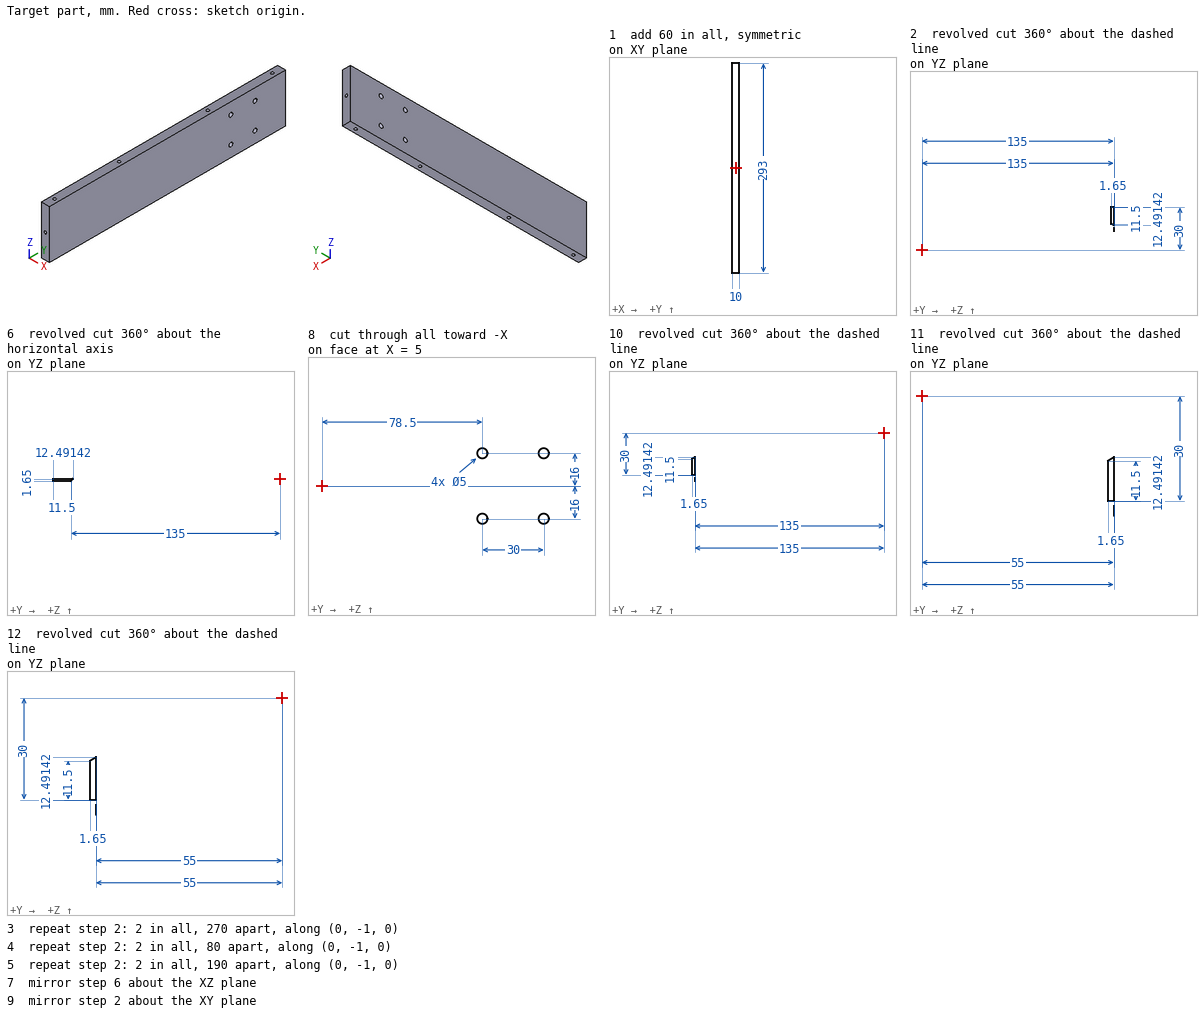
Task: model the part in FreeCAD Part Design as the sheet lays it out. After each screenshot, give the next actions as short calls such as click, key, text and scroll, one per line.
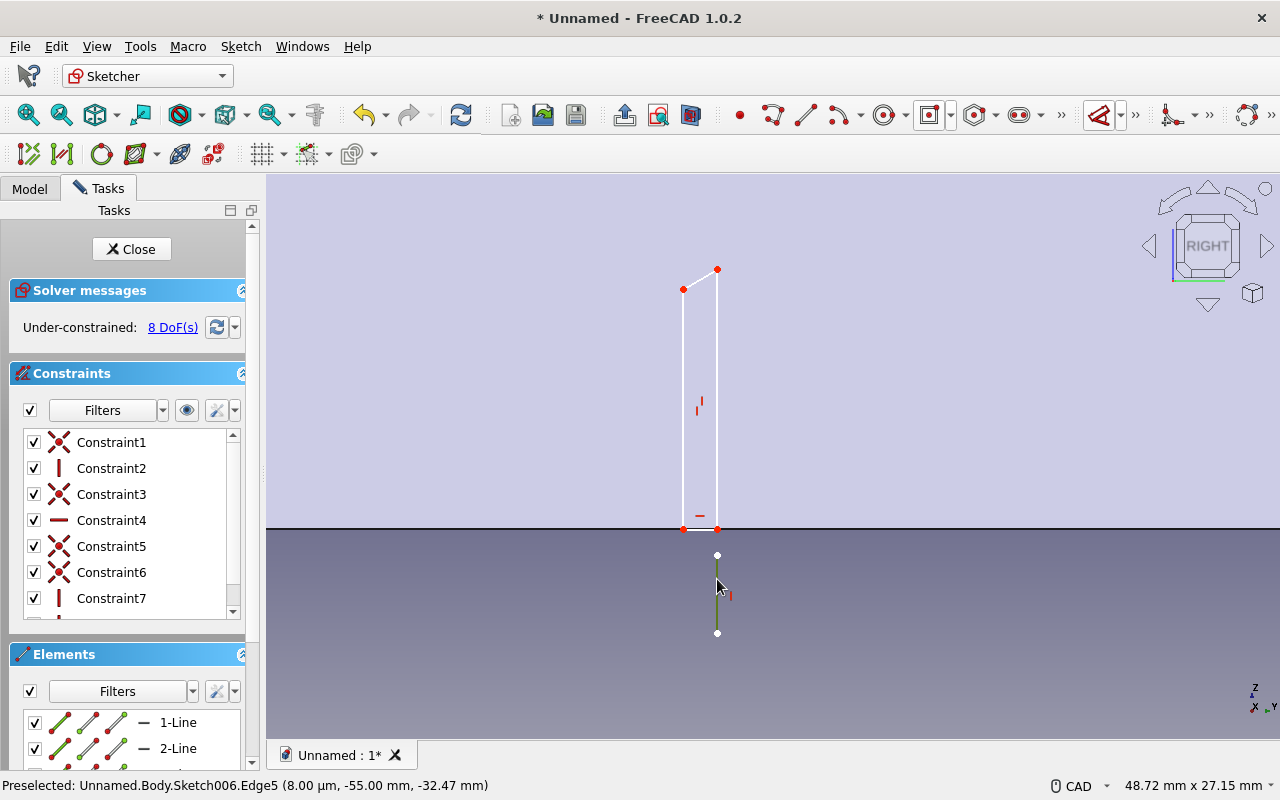
key(g)
key(n)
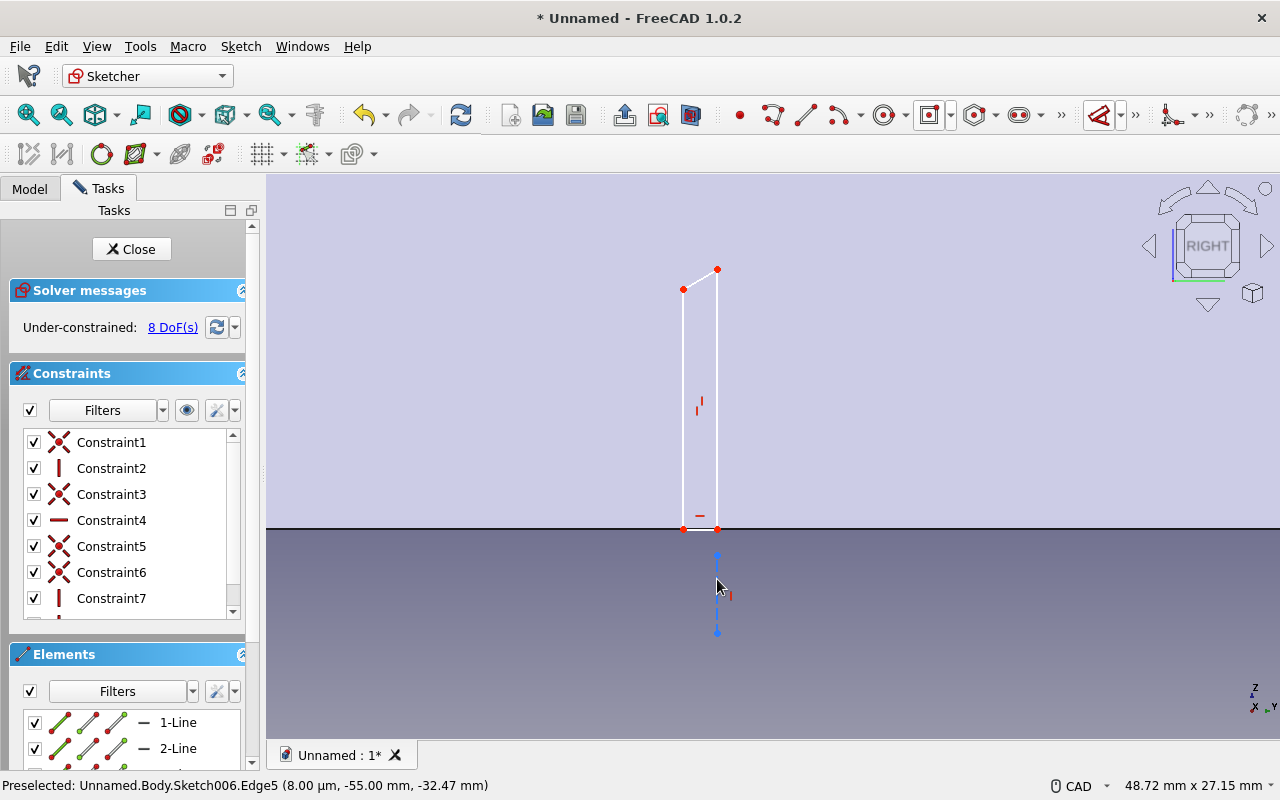
click(717, 270)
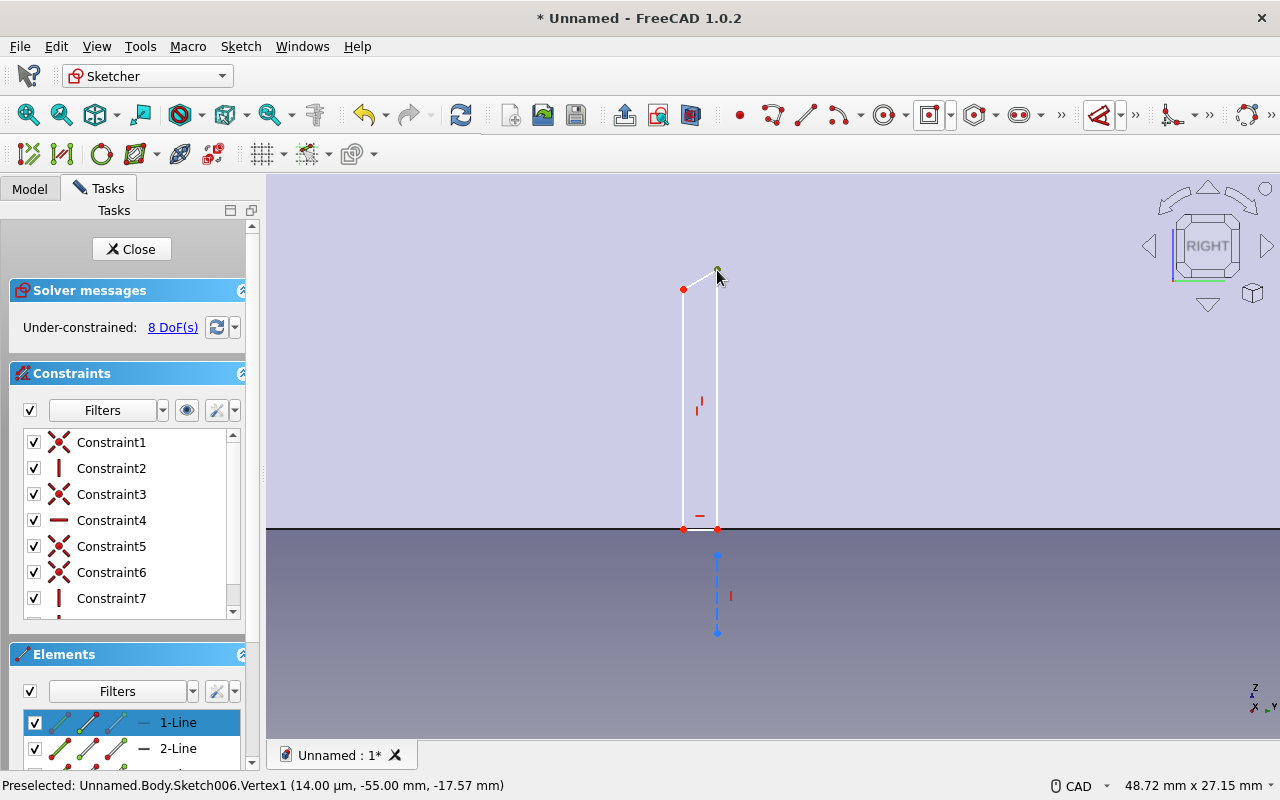
click(1120, 116)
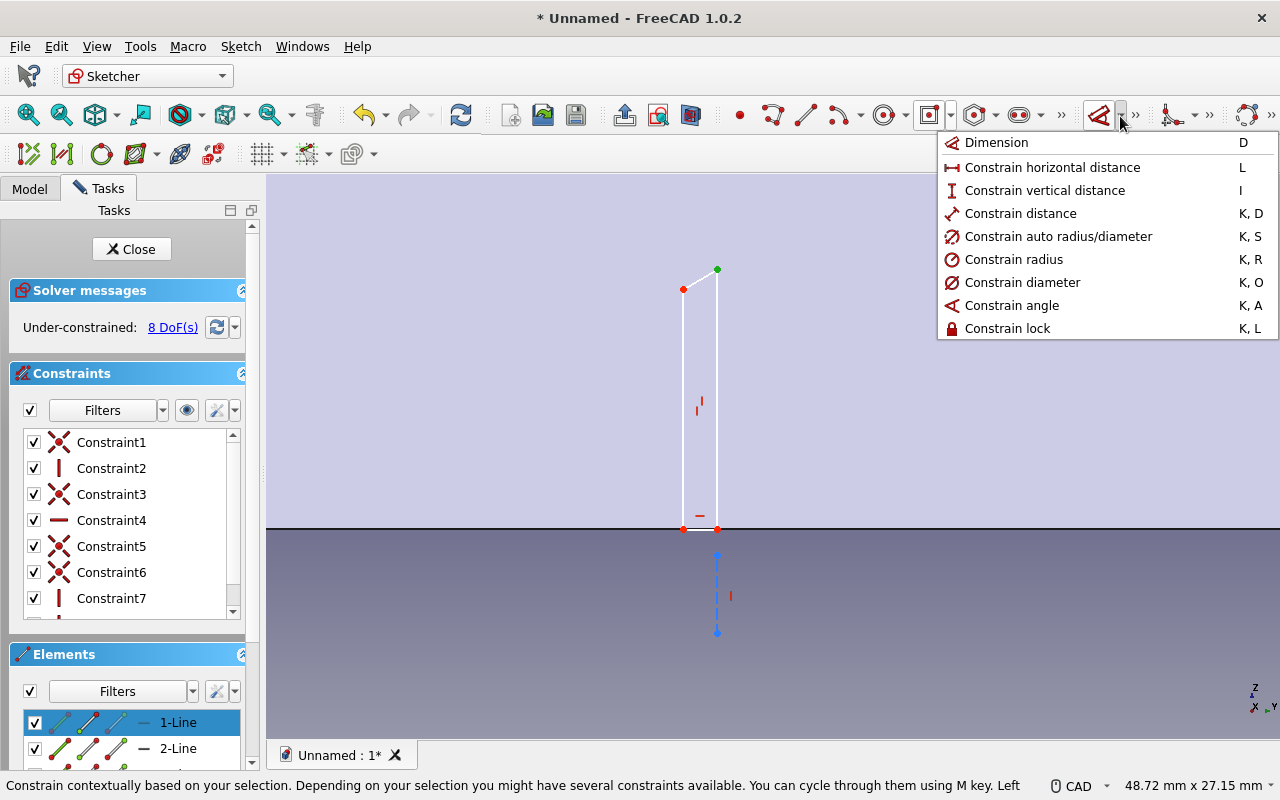
click(1108, 168)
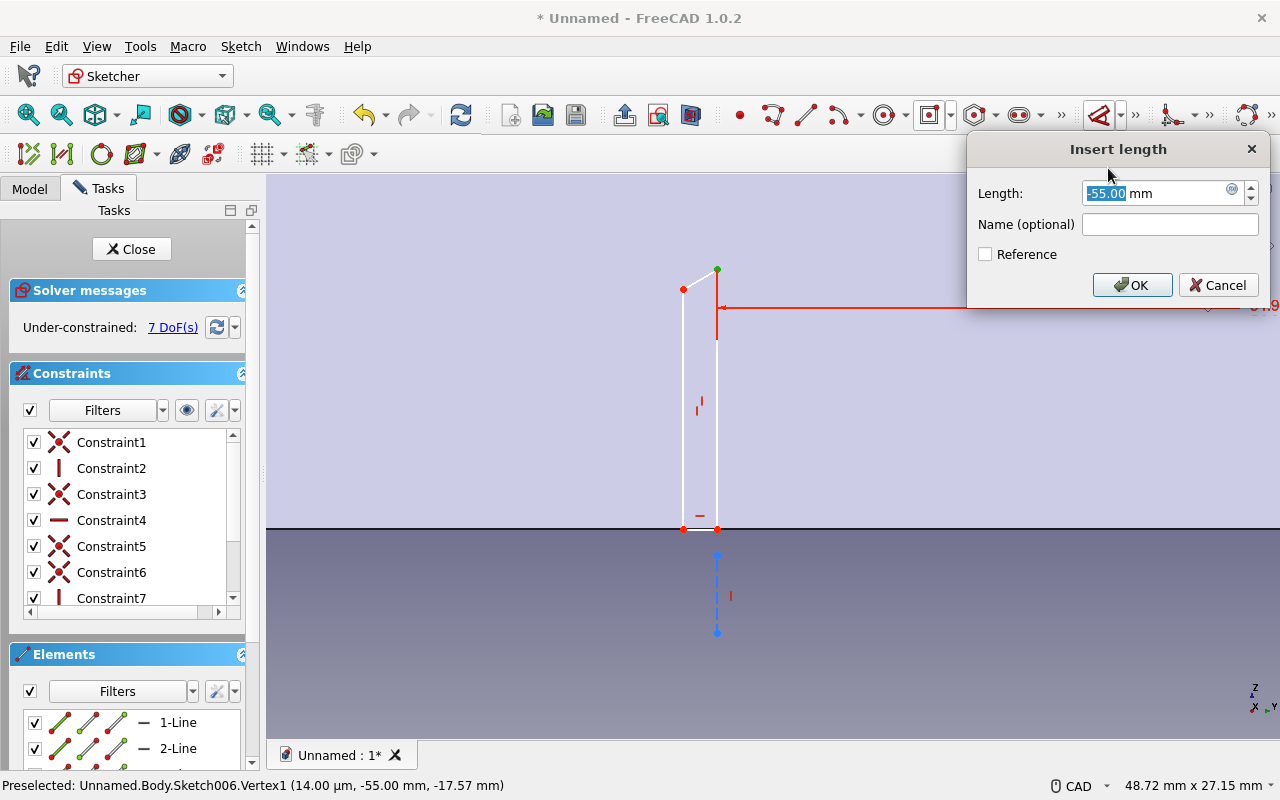
text(-55)
key(Return)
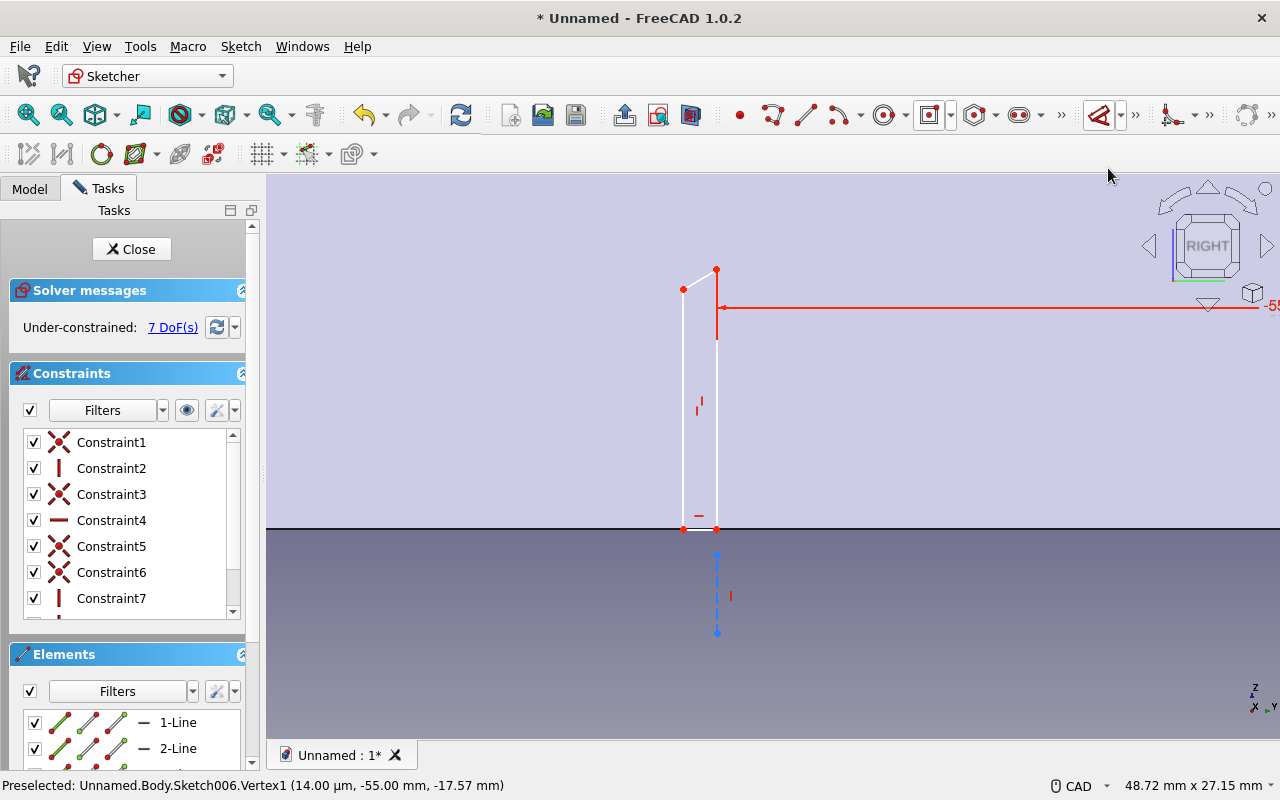
click(683, 530)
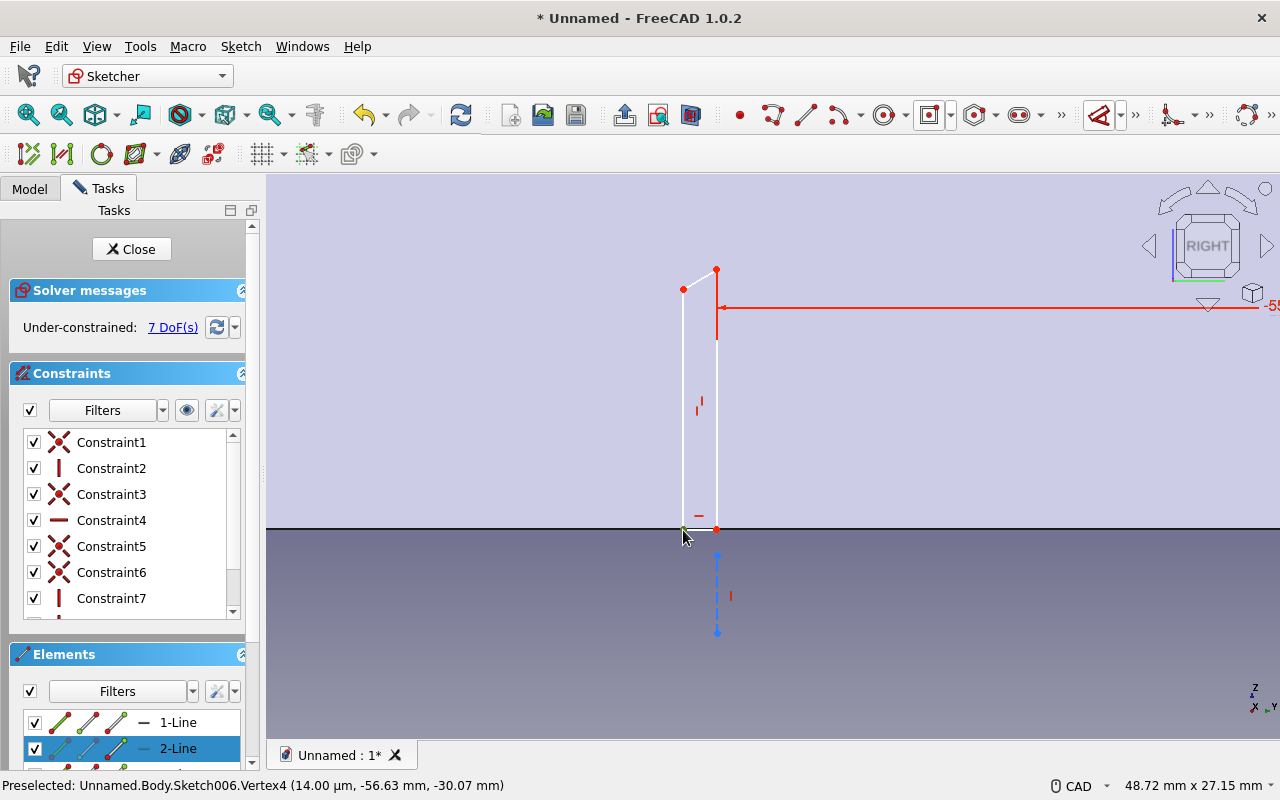
click(1120, 116)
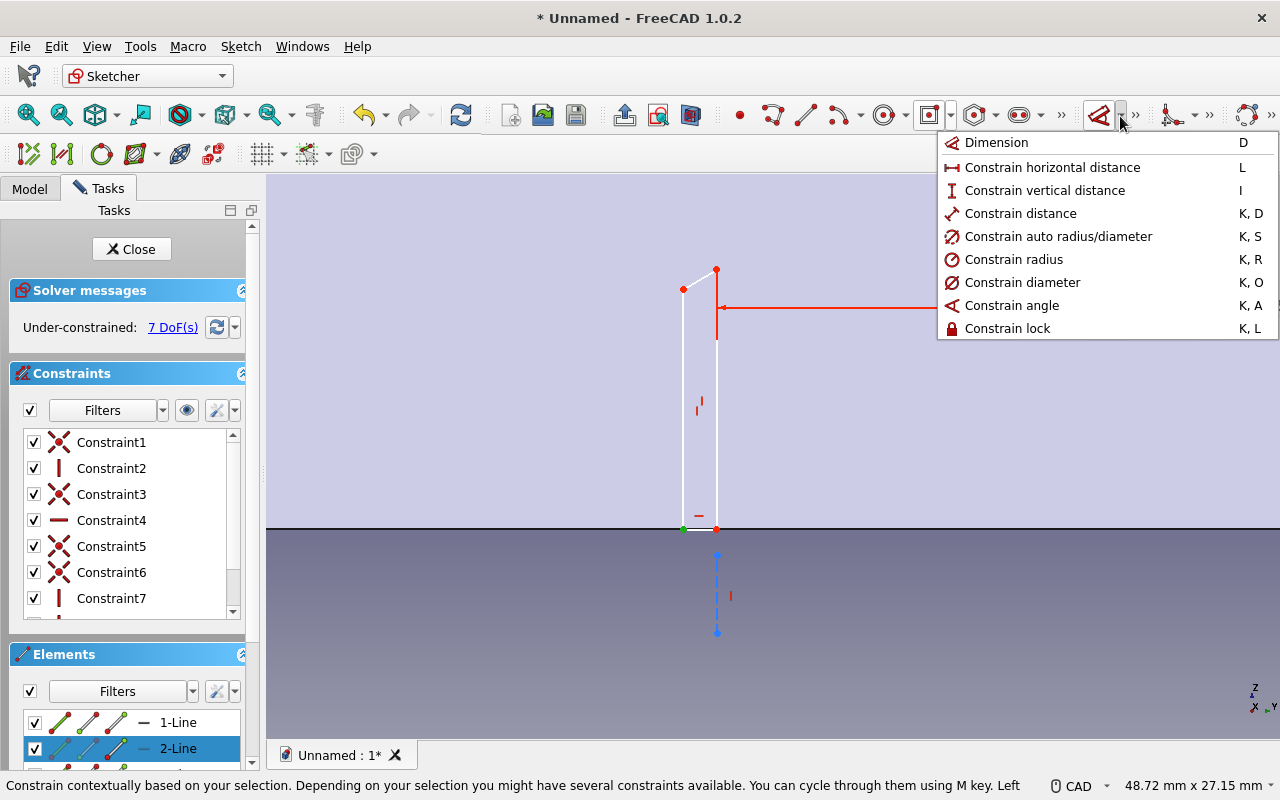
click(1108, 190)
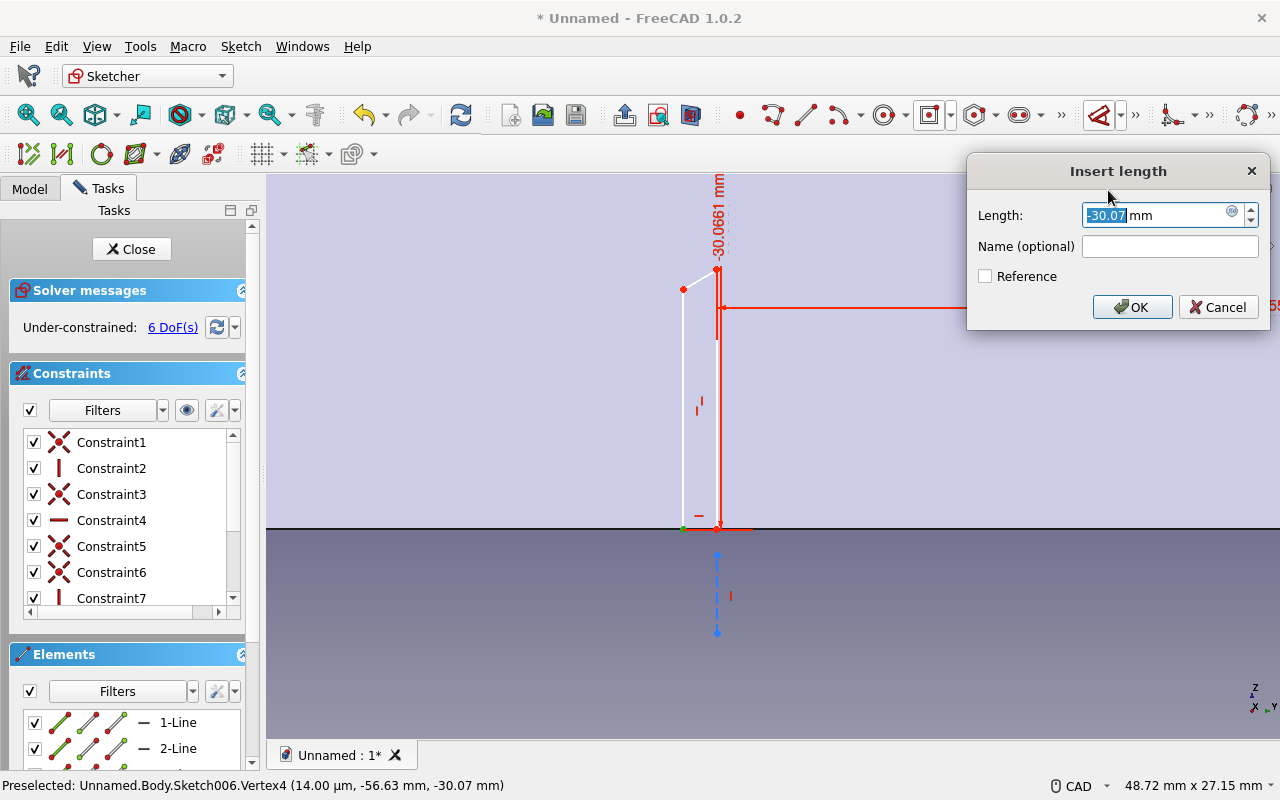
text(-30)
key(Return)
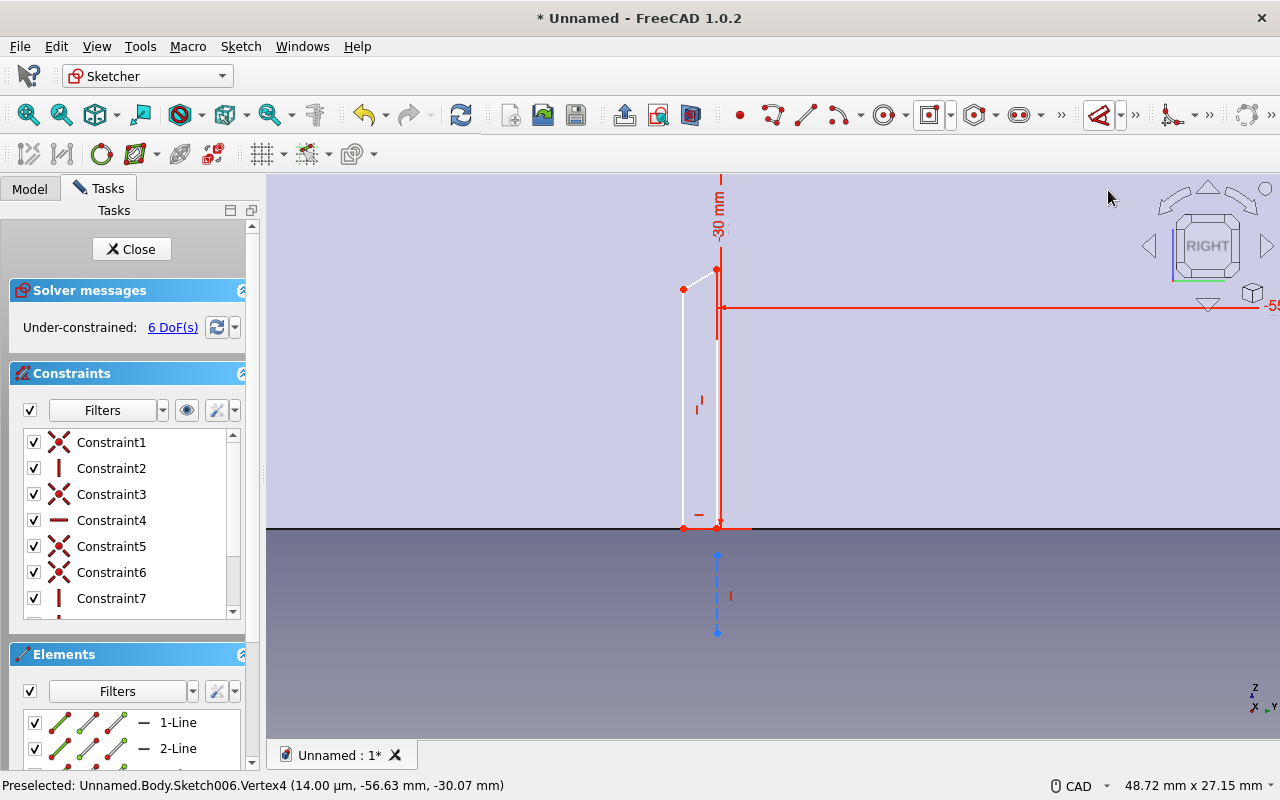
click(717, 556)